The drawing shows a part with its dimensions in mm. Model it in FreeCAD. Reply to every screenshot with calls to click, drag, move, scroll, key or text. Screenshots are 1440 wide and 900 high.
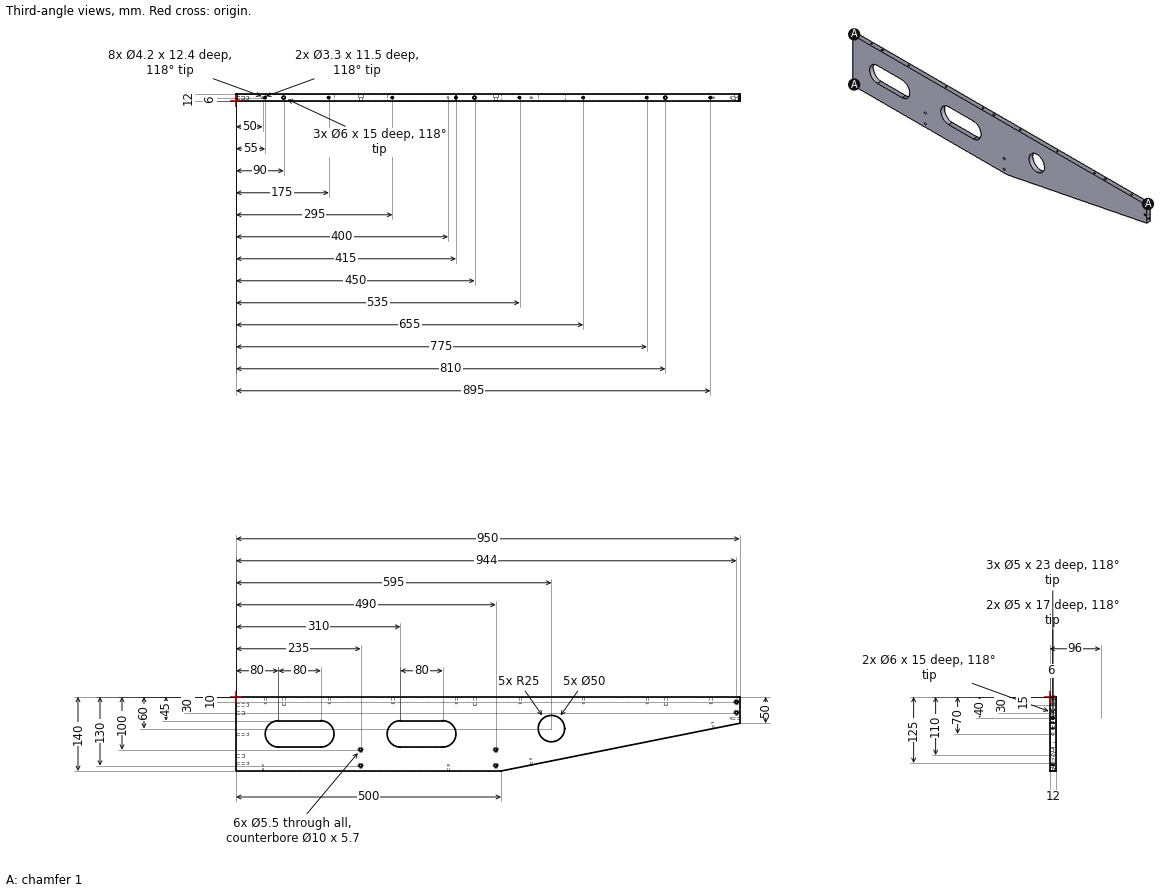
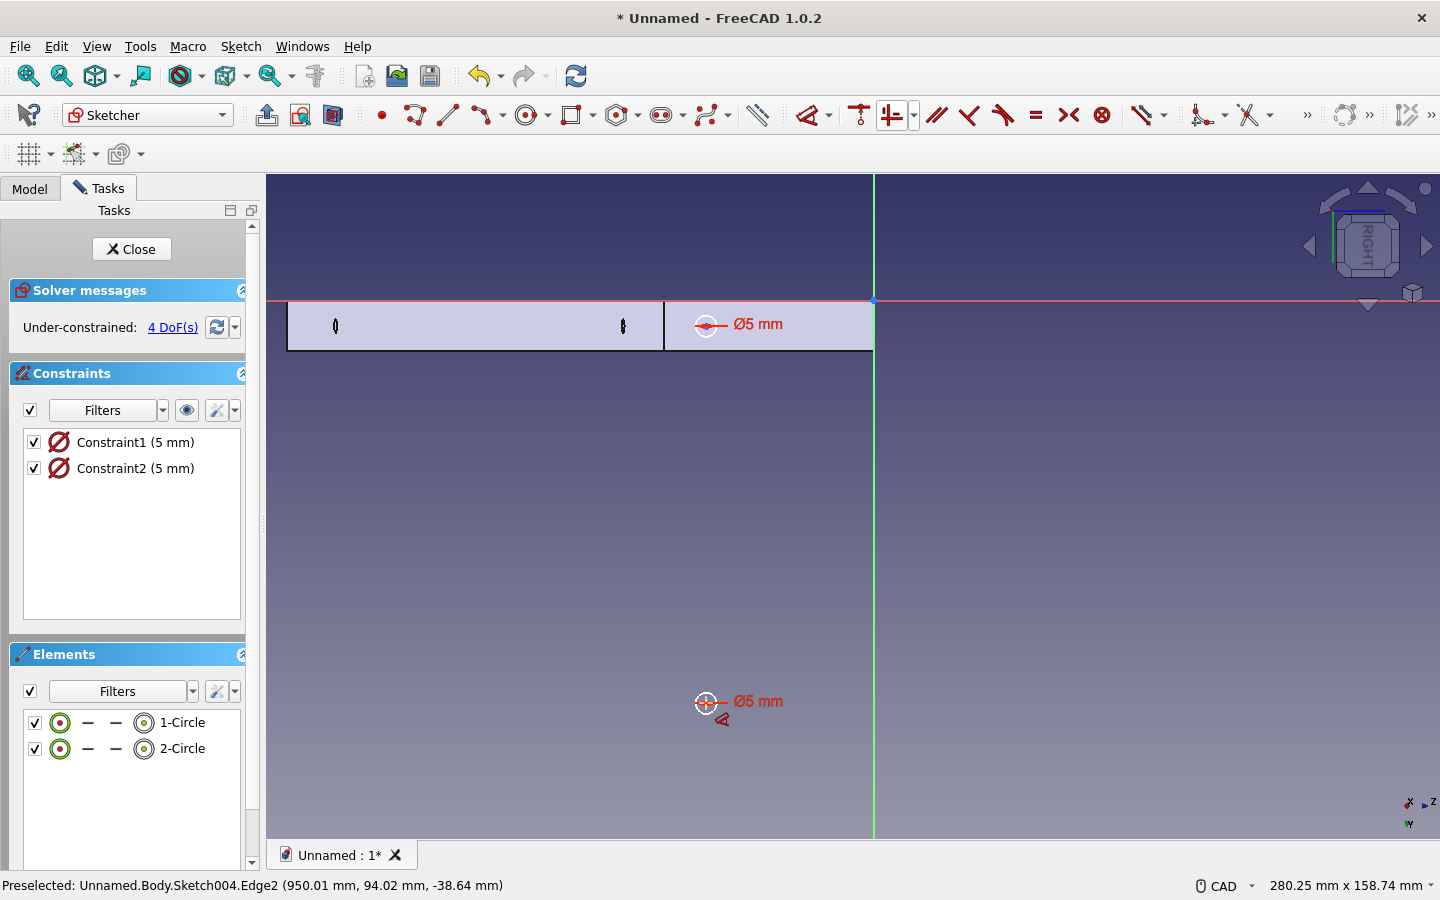
scroll(706, 326, up, 3)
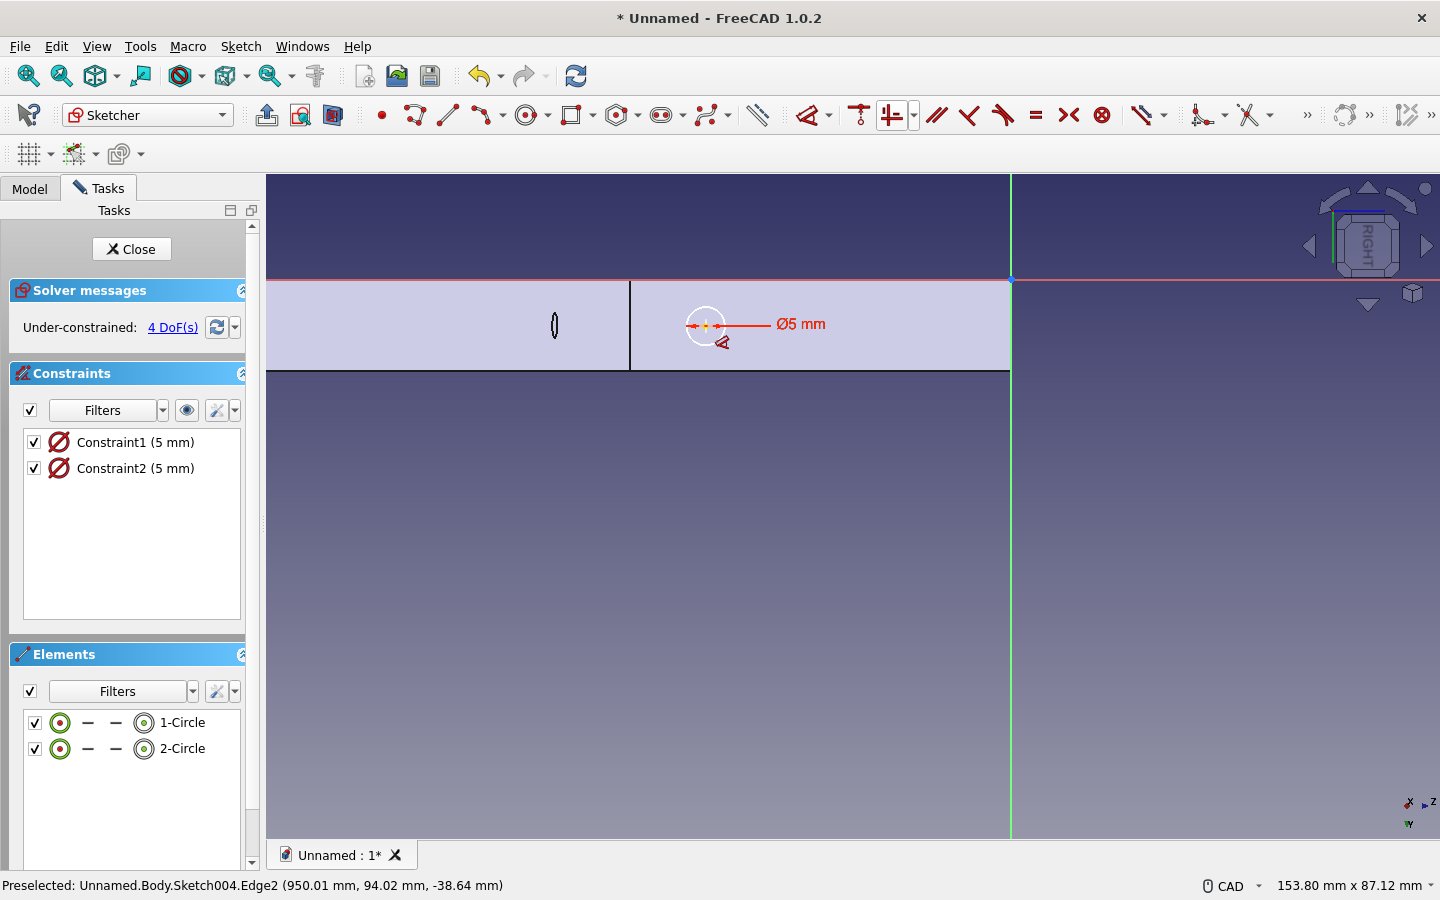
click(706, 326)
click(1045, 303)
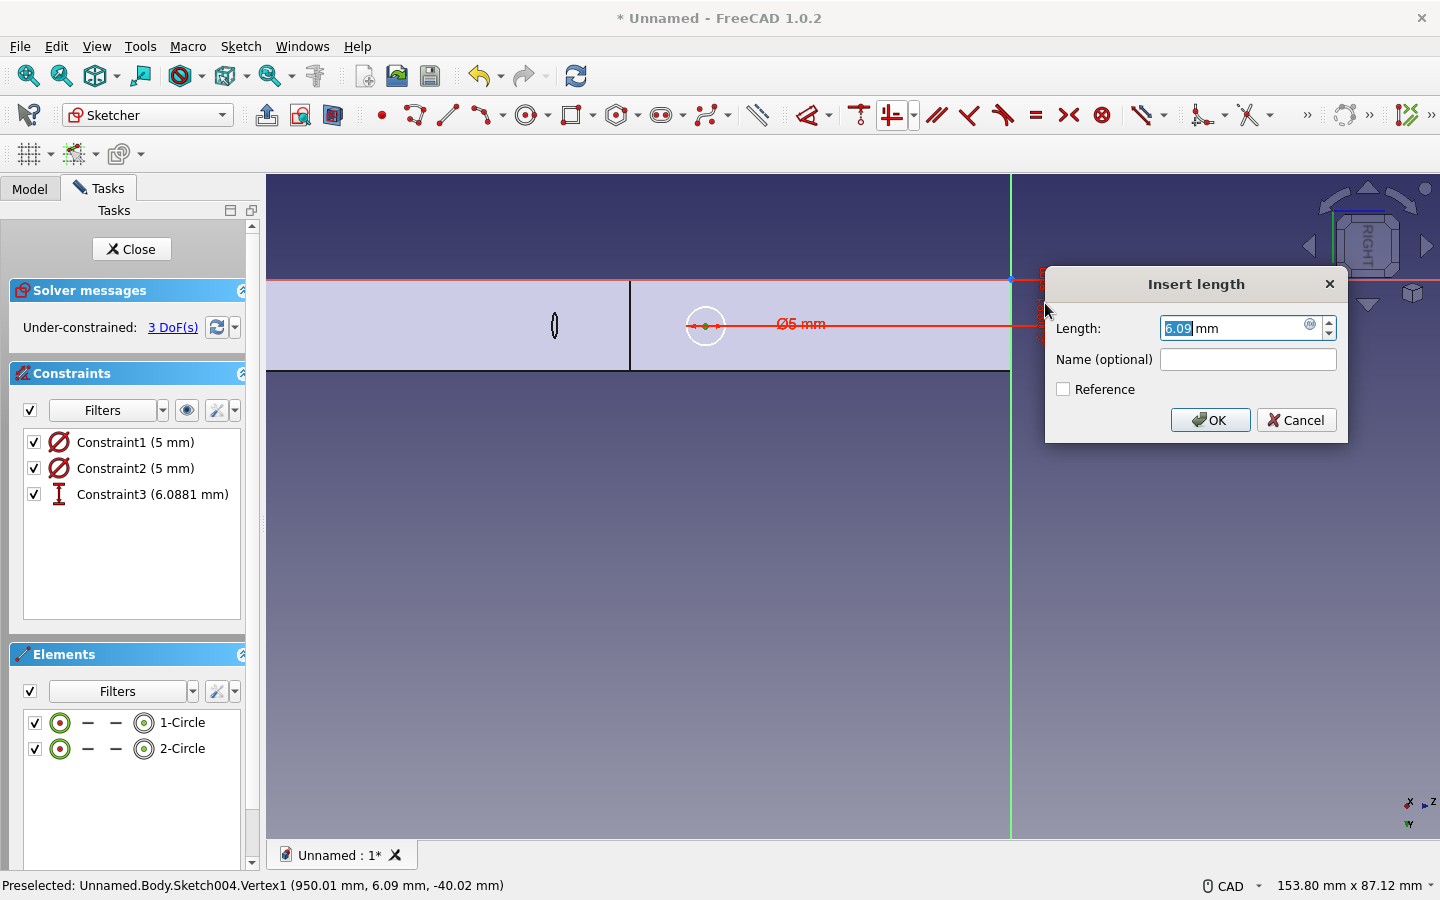
text(6)
key(Return)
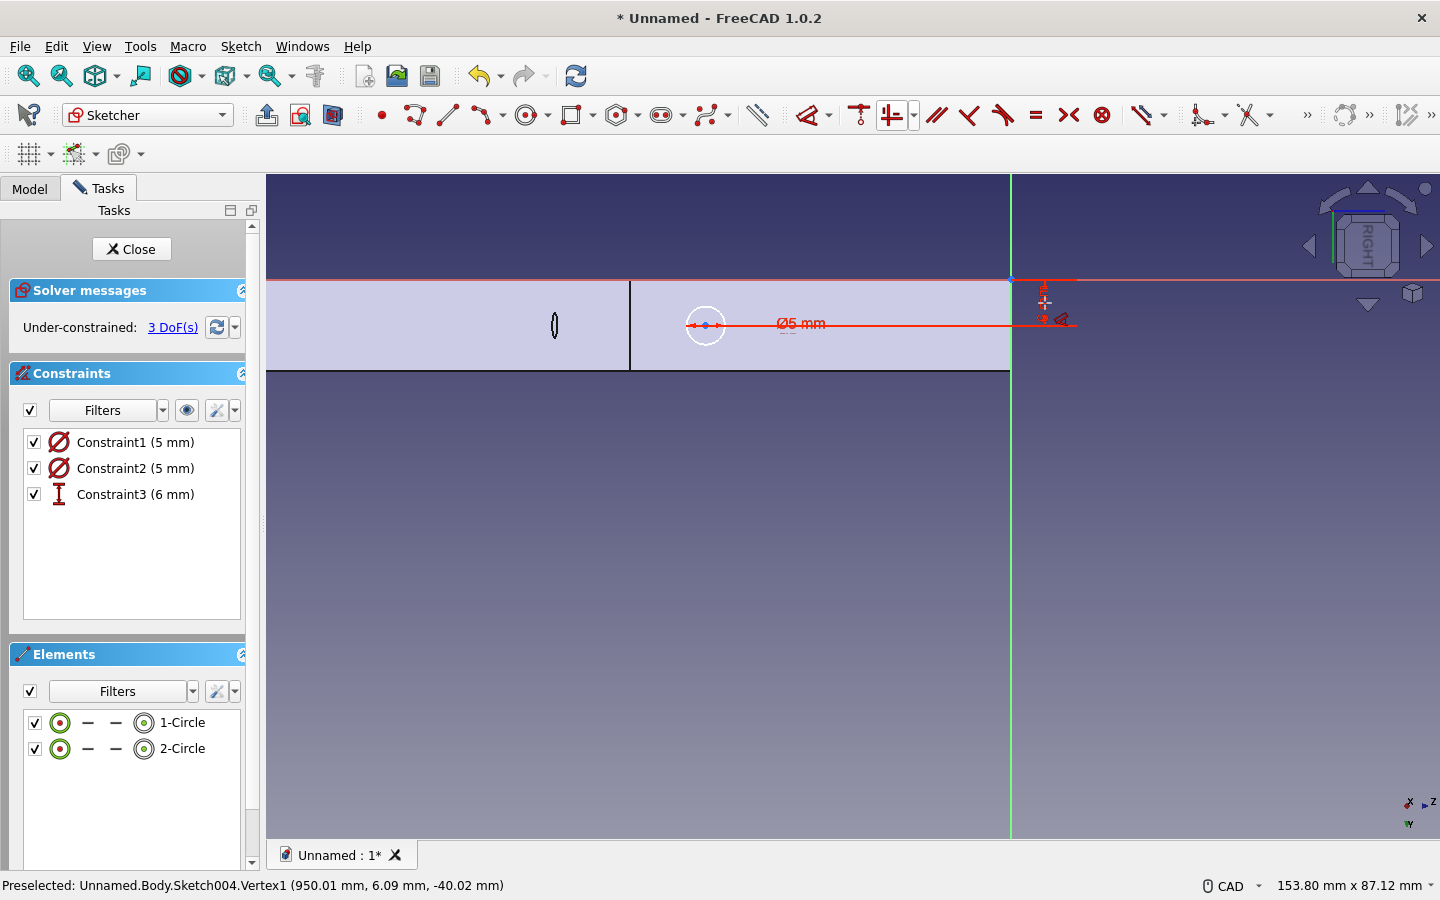
click(706, 326)
click(859, 246)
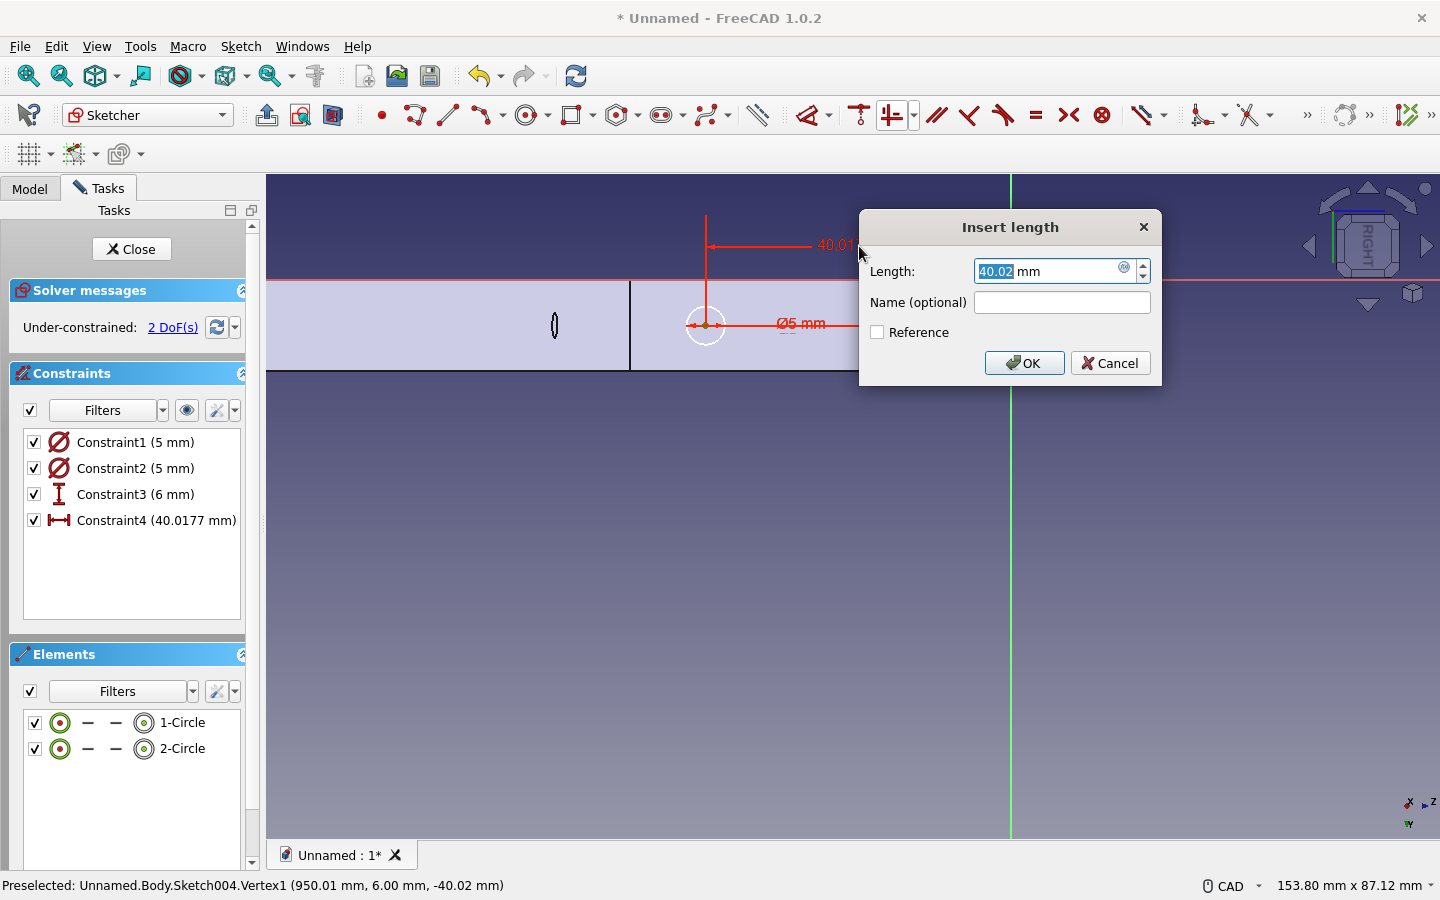
text(40)
key(Return)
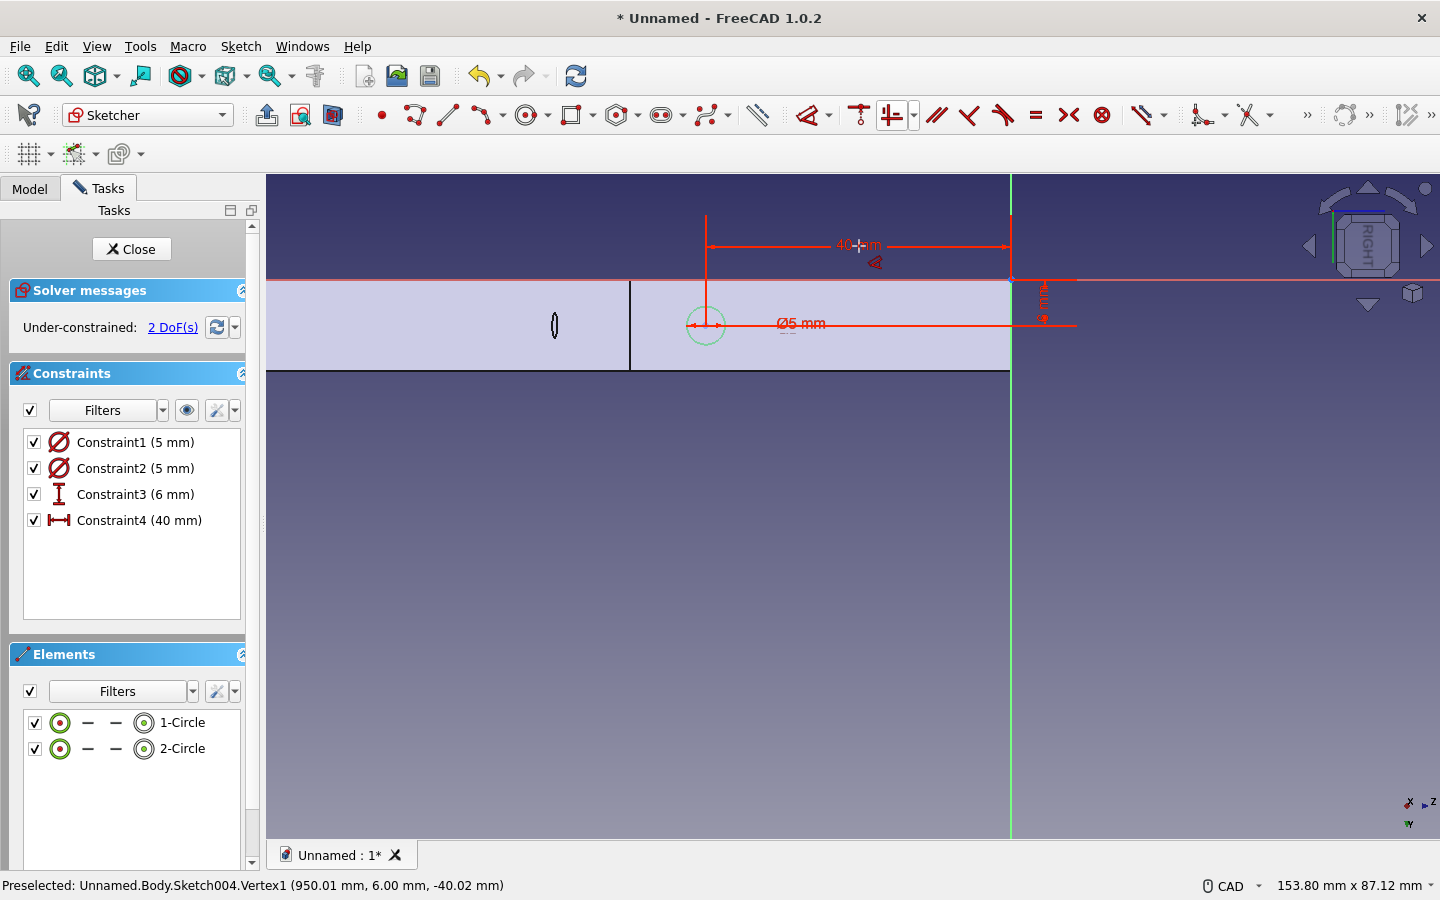
scroll(706, 325, down, 3)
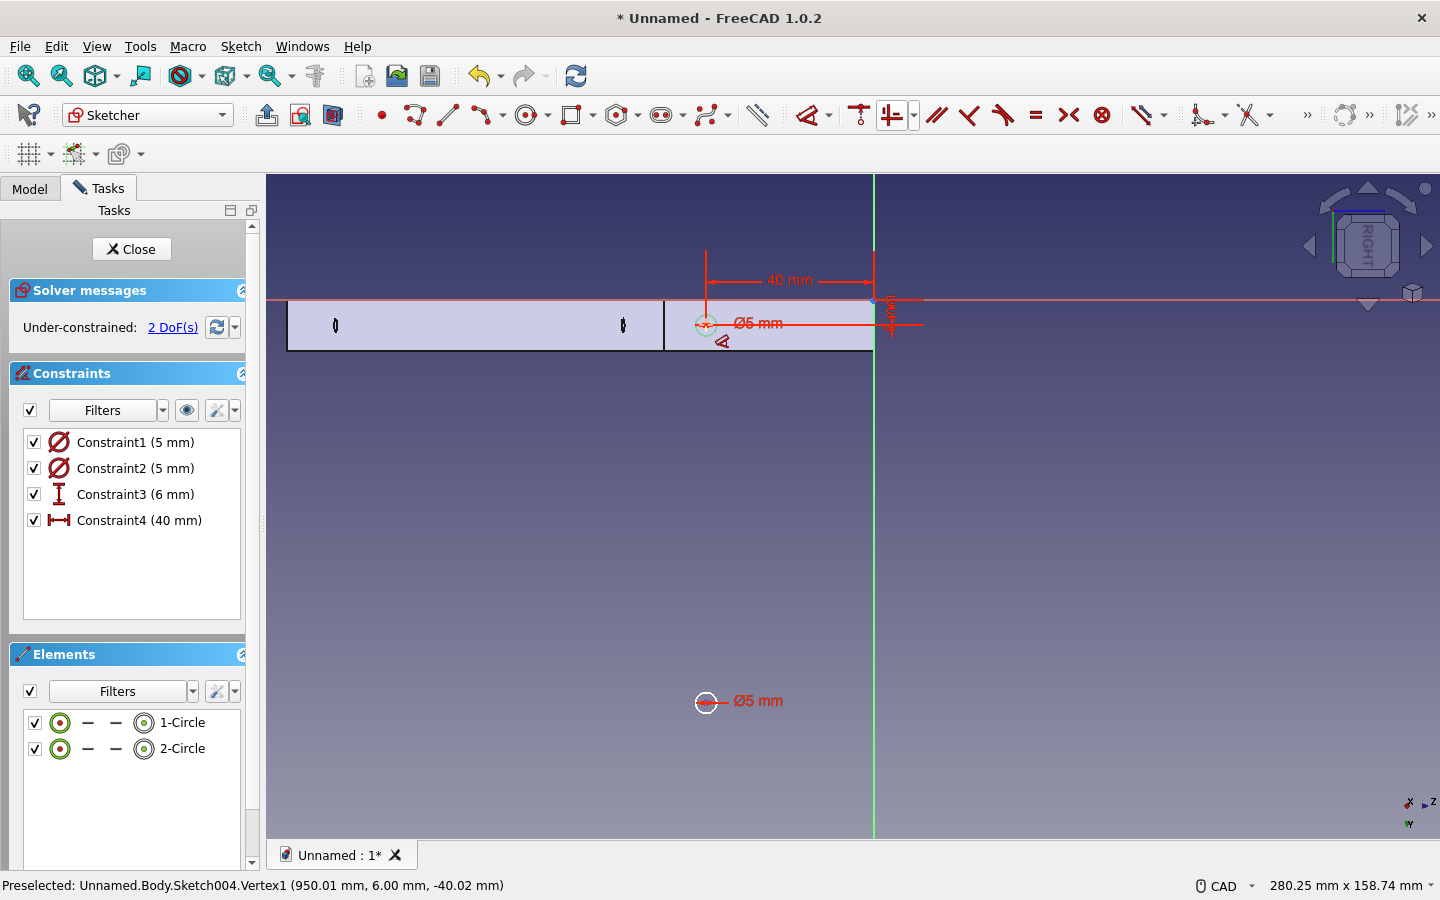
click(706, 703)
click(790, 737)